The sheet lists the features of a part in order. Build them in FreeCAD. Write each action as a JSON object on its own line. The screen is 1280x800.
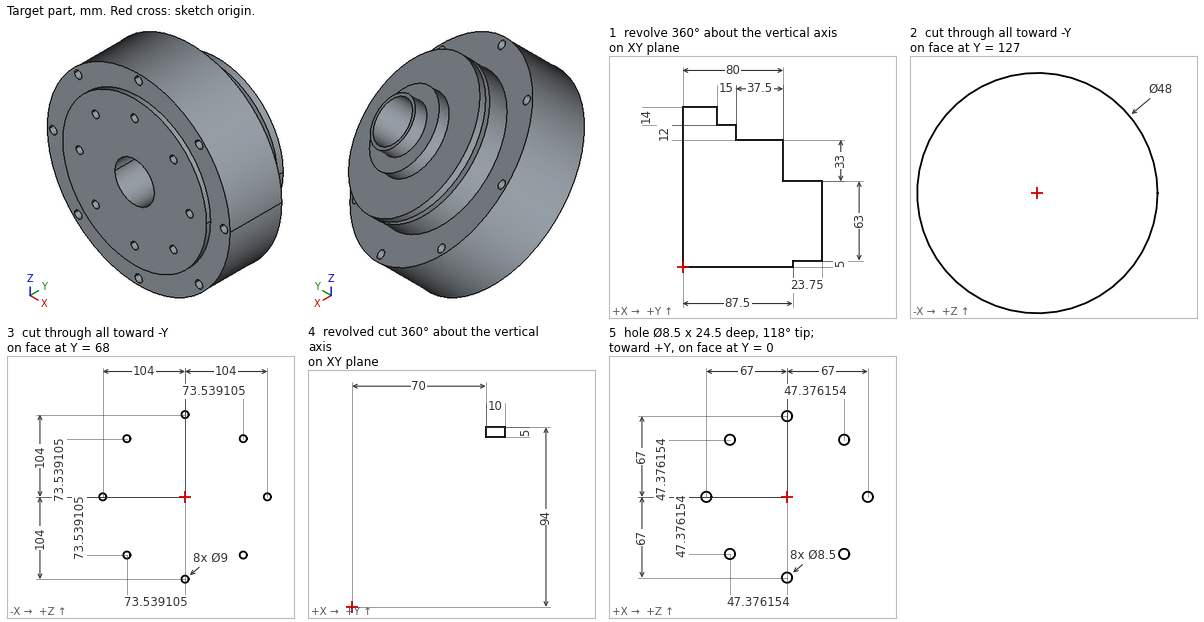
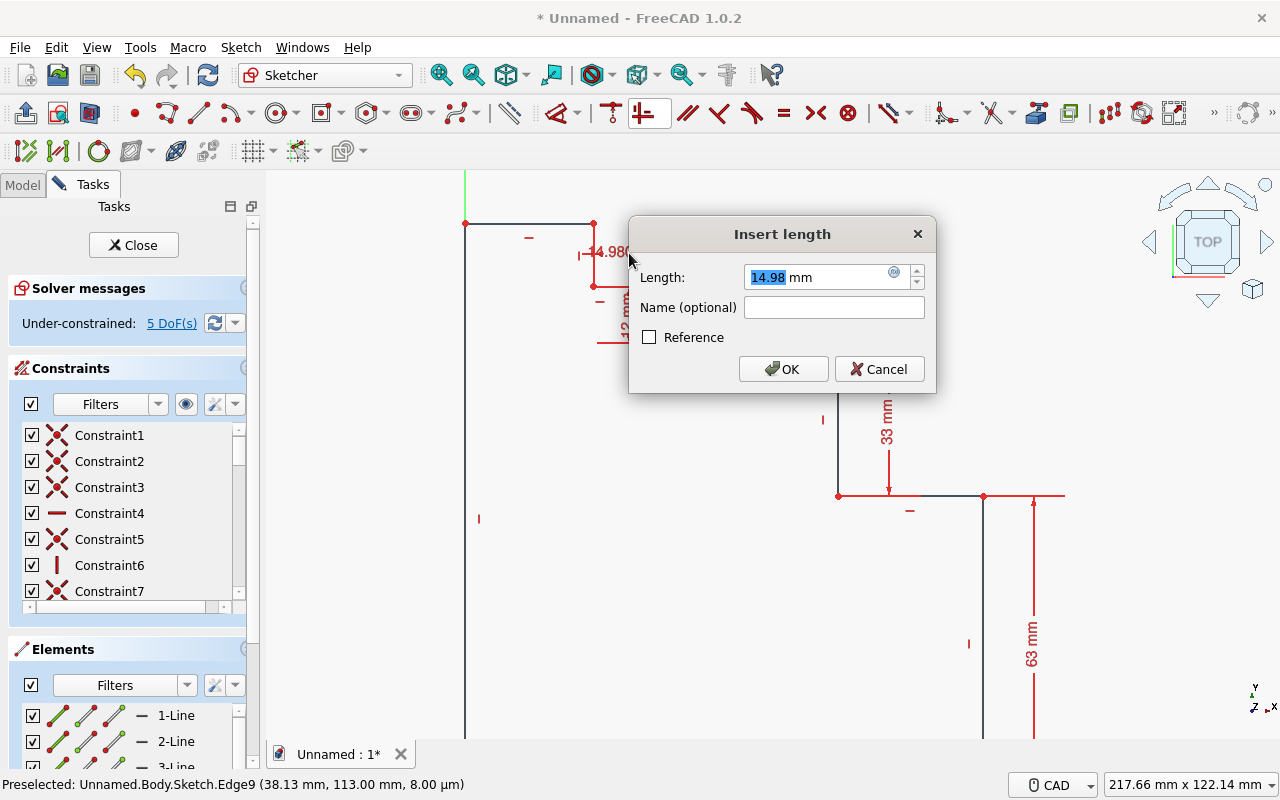
{"action": "type", "text": "15"}
{"action": "key", "text": "Return"}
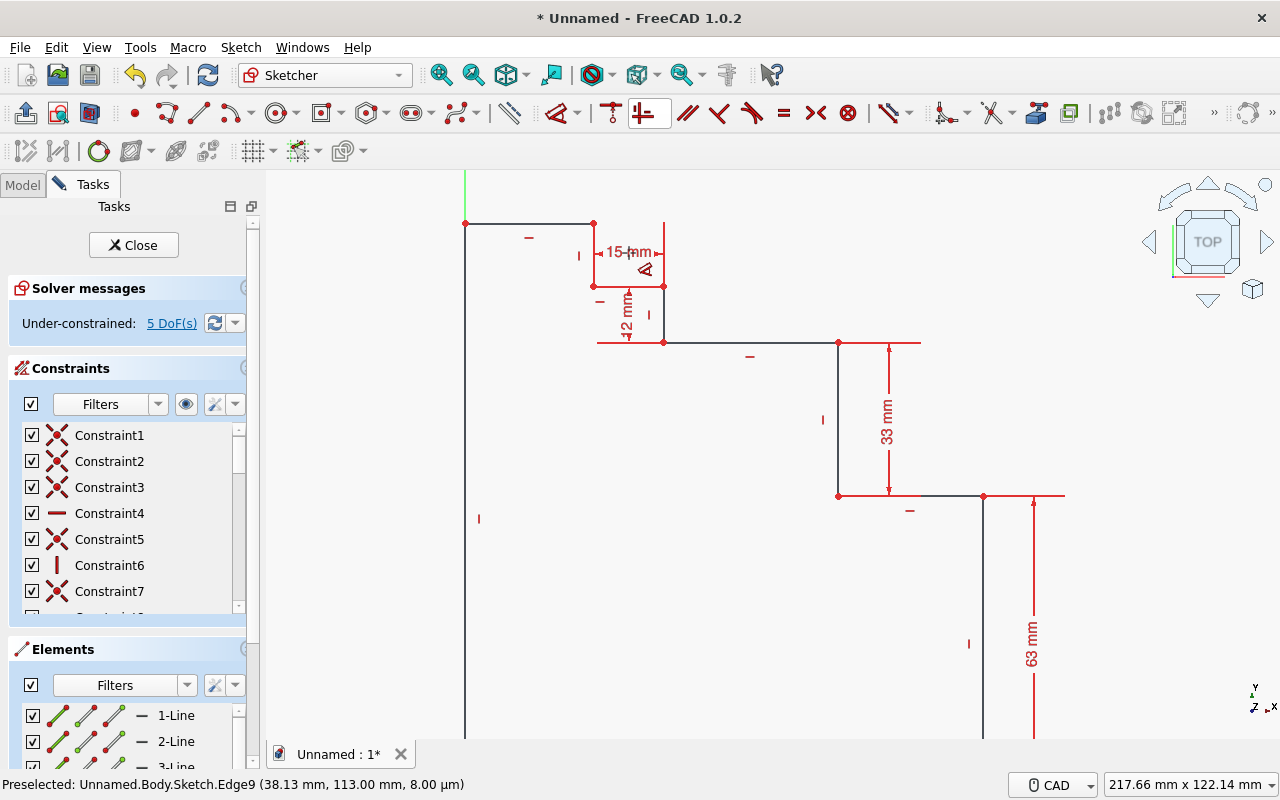
{"action": "left_click", "coordinate": [594, 268]}
{"action": "left_click", "coordinate": [560, 277]}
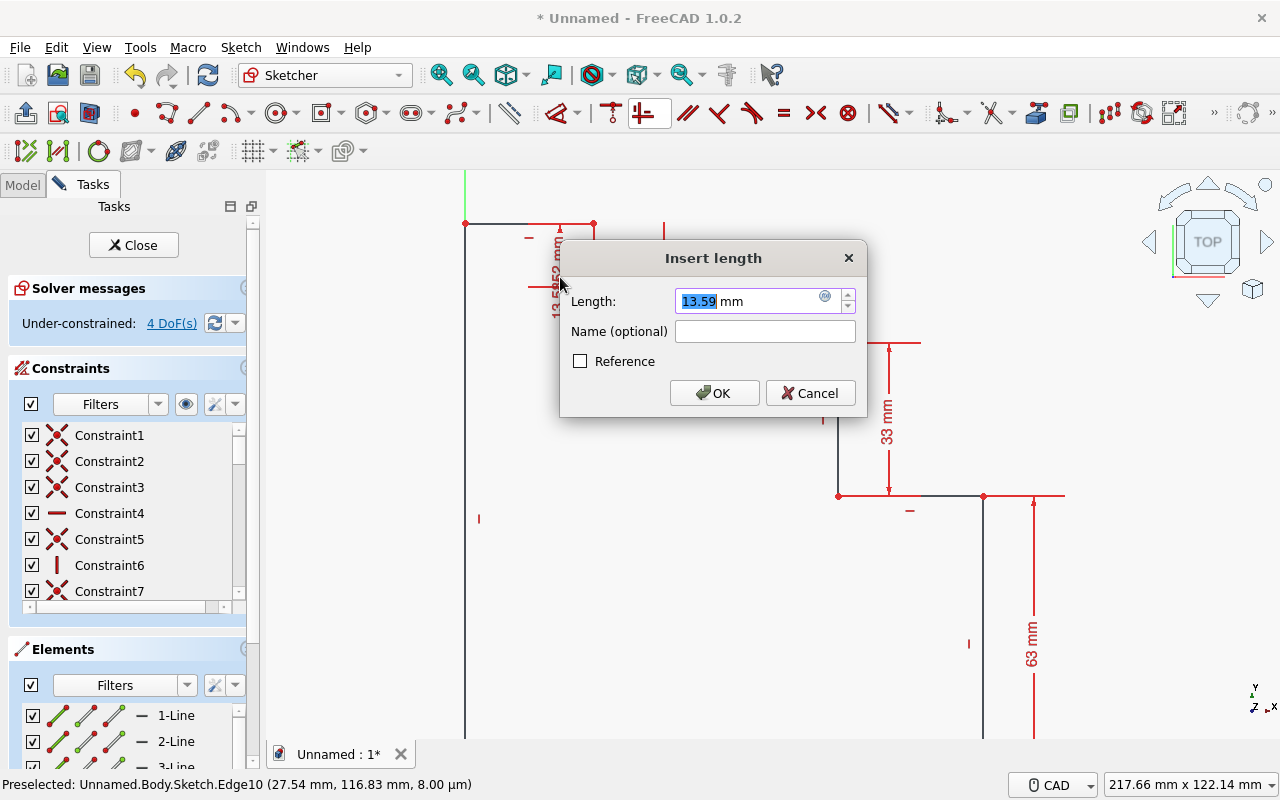
{"action": "type", "text": "14"}
{"action": "key", "text": "Return"}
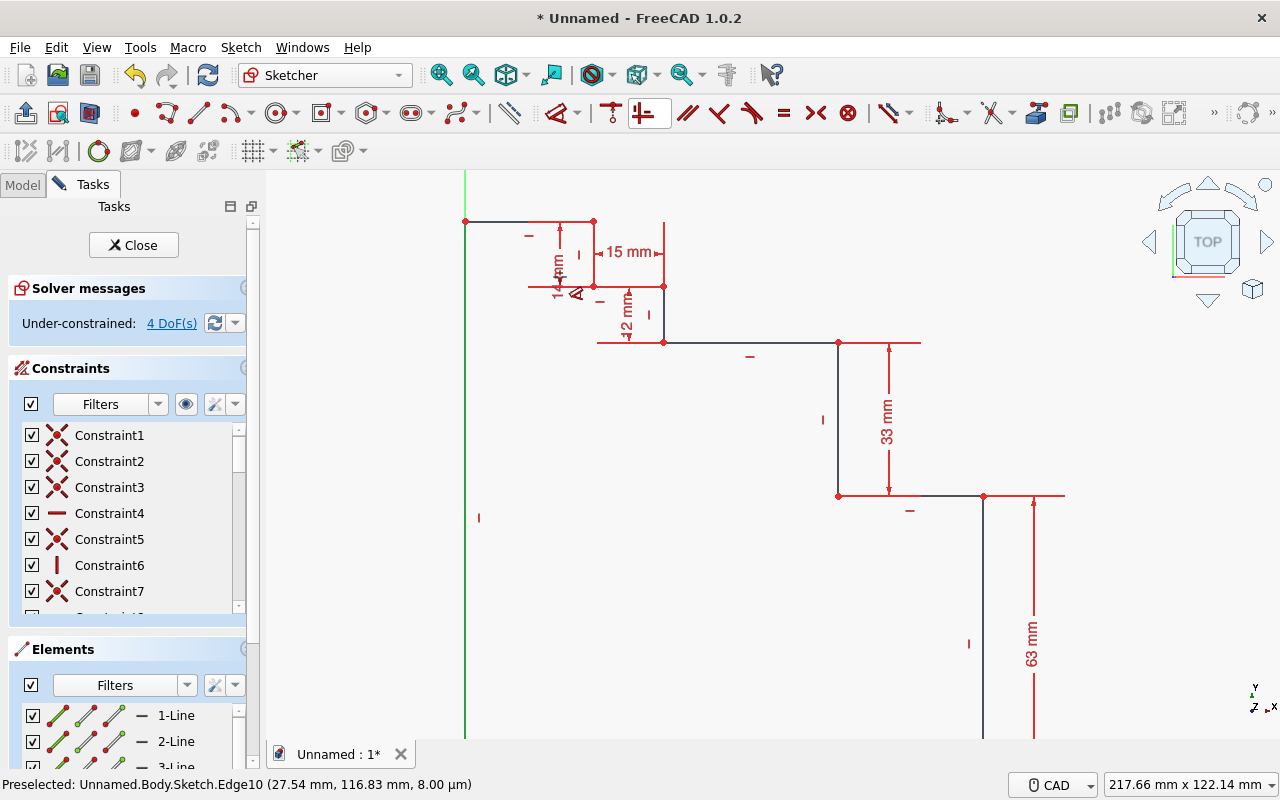
{"action": "left_click", "coordinate": [838, 496]}
{"action": "left_click", "coordinate": [652, 462]}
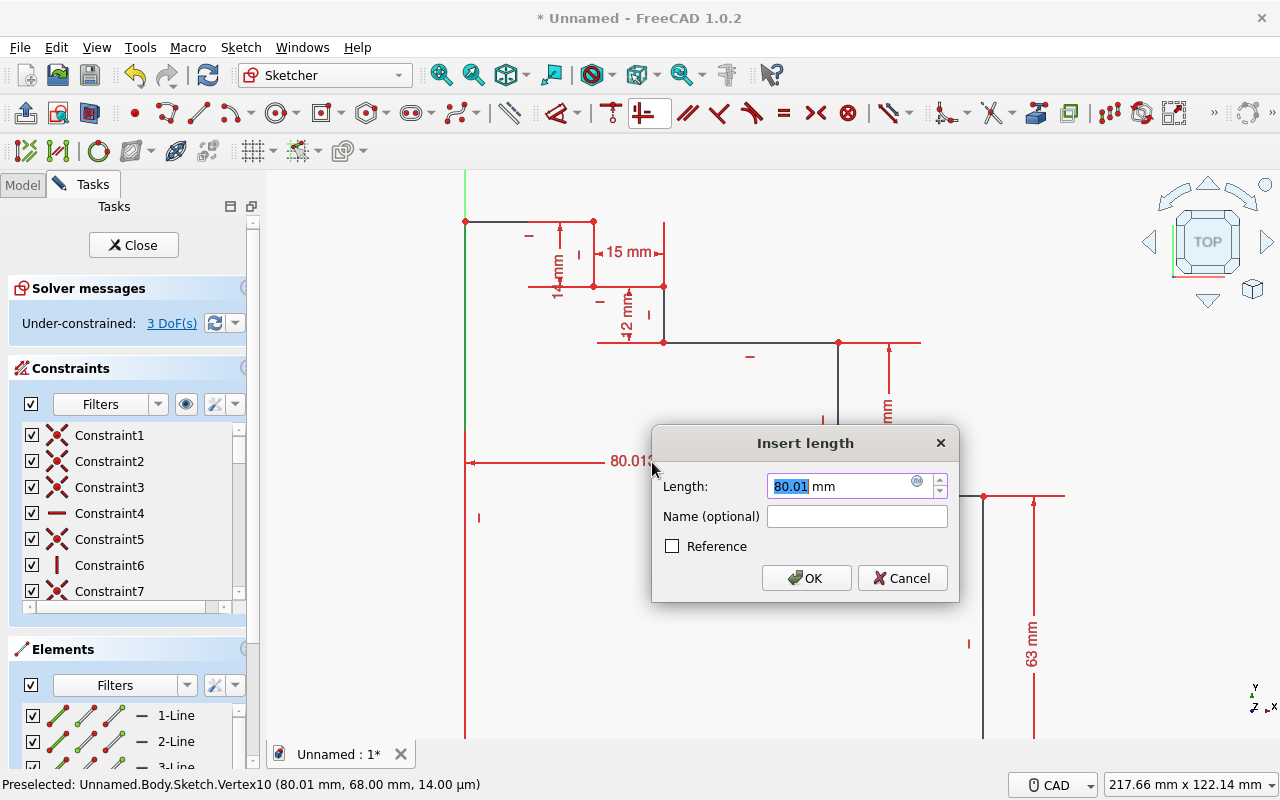
{"action": "type", "text": "80"}
{"action": "key", "text": "Return"}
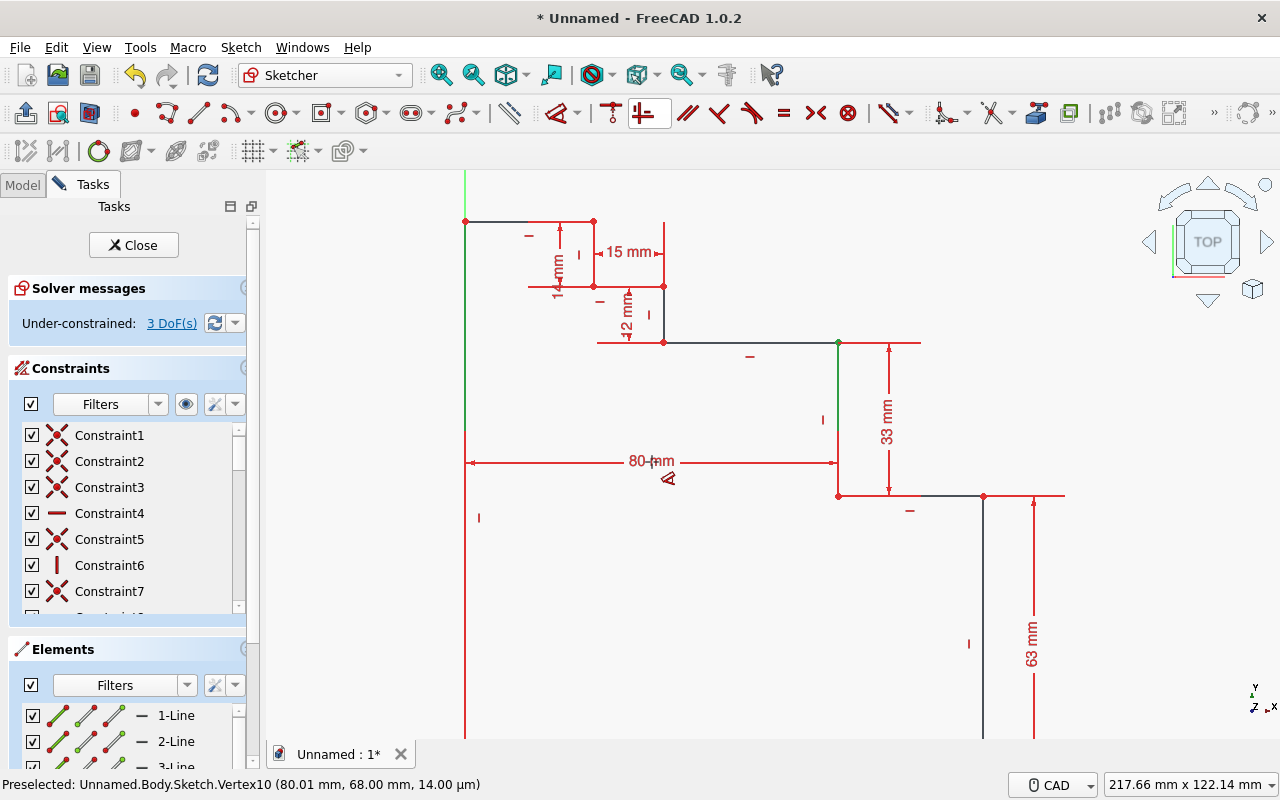
{"action": "scroll", "coordinate": [664, 326], "scroll_direction": "down", "scroll_amount": 2}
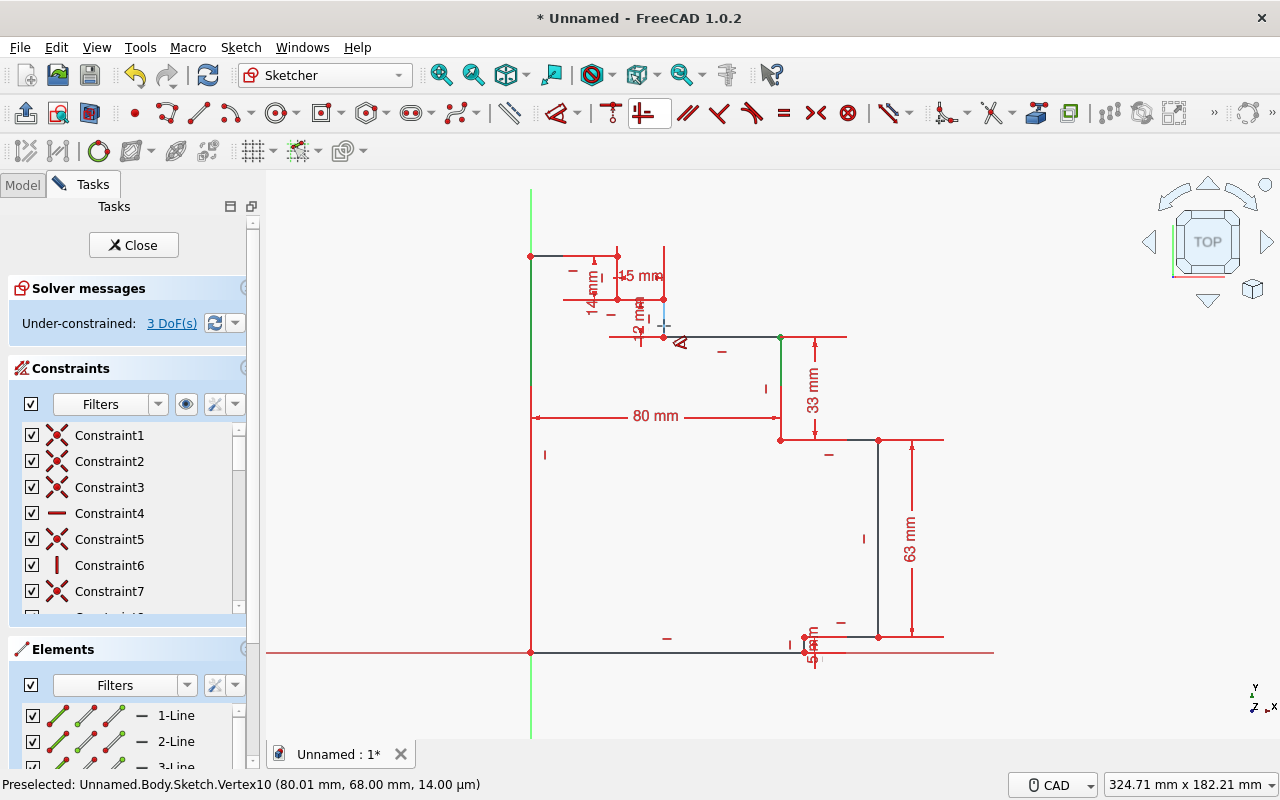
{"action": "left_click", "coordinate": [613, 653]}
{"action": "left_click", "coordinate": [668, 687]}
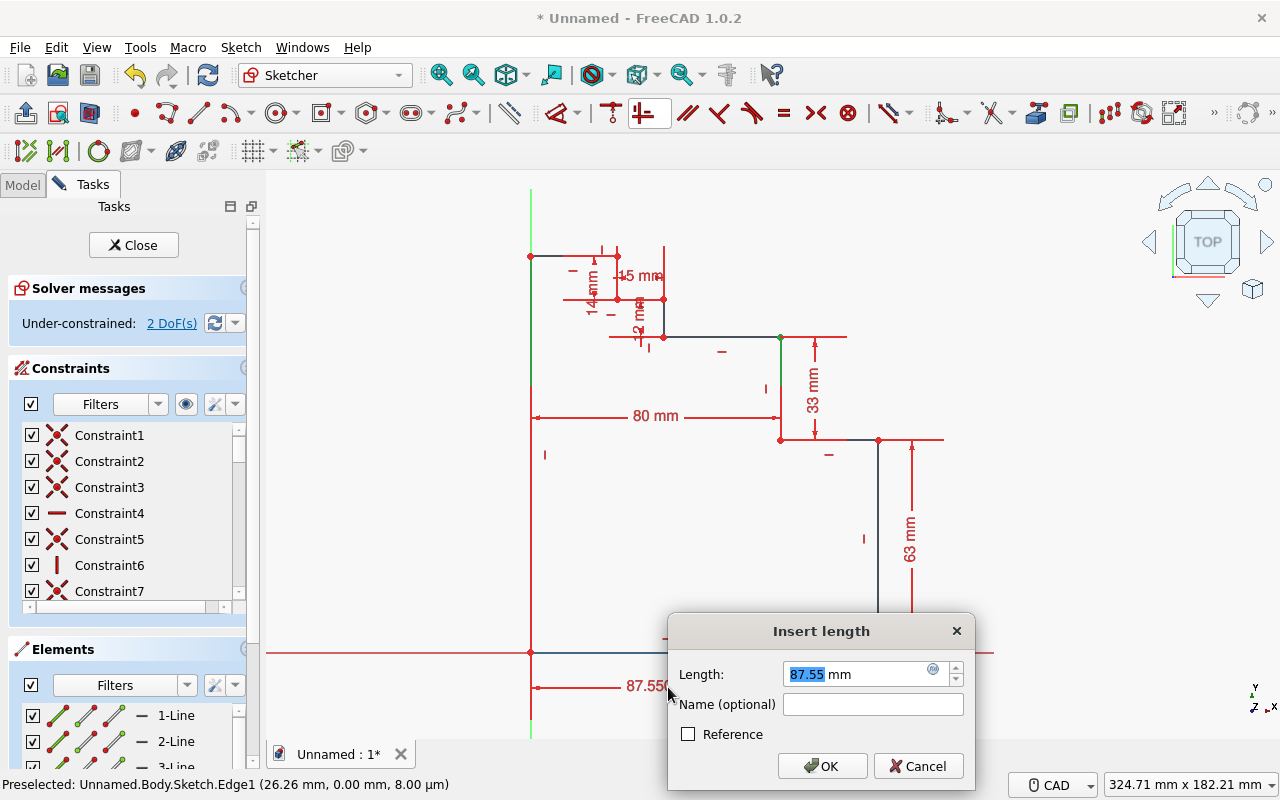
{"action": "type", "text": "87.5"}
{"action": "key", "text": "Return"}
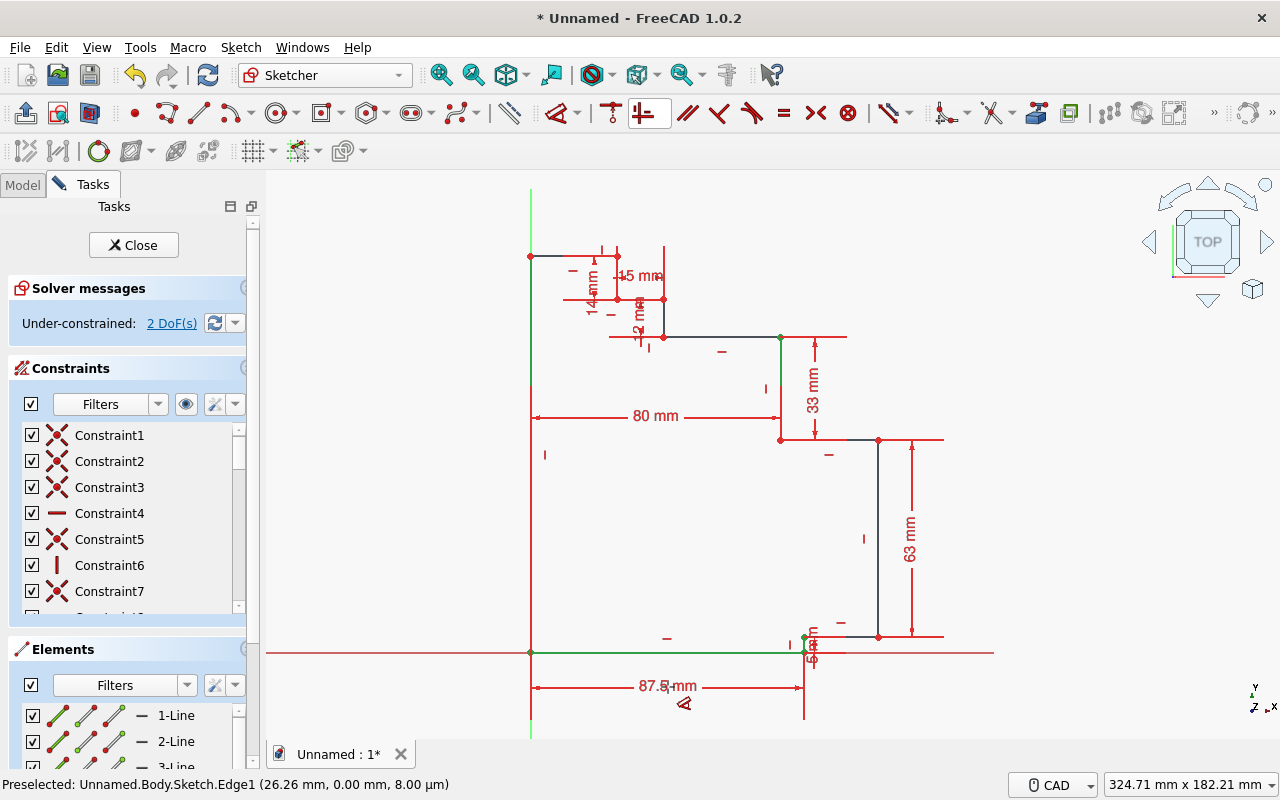
{"action": "left_click", "coordinate": [746, 337]}
{"action": "left_click", "coordinate": [722, 303]}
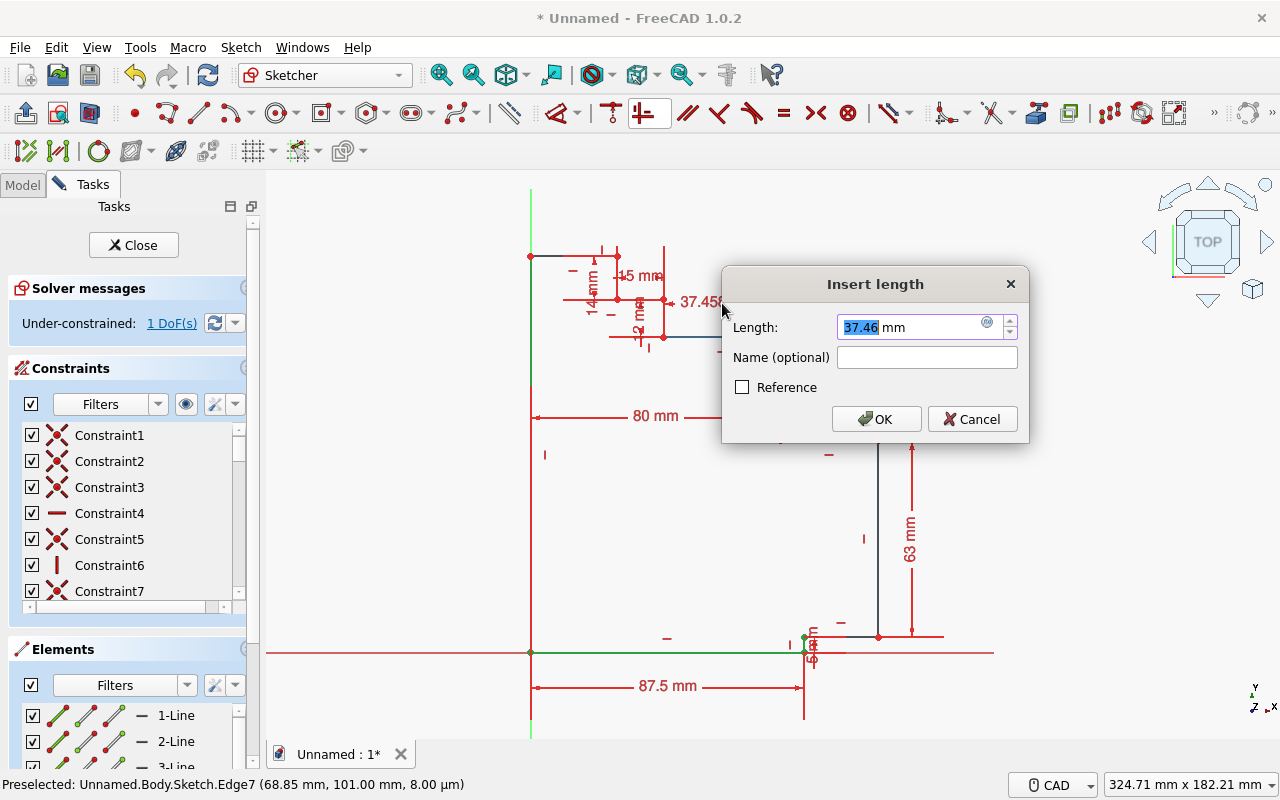
{"action": "type", "text": "37.5"}
{"action": "key", "text": "Return"}